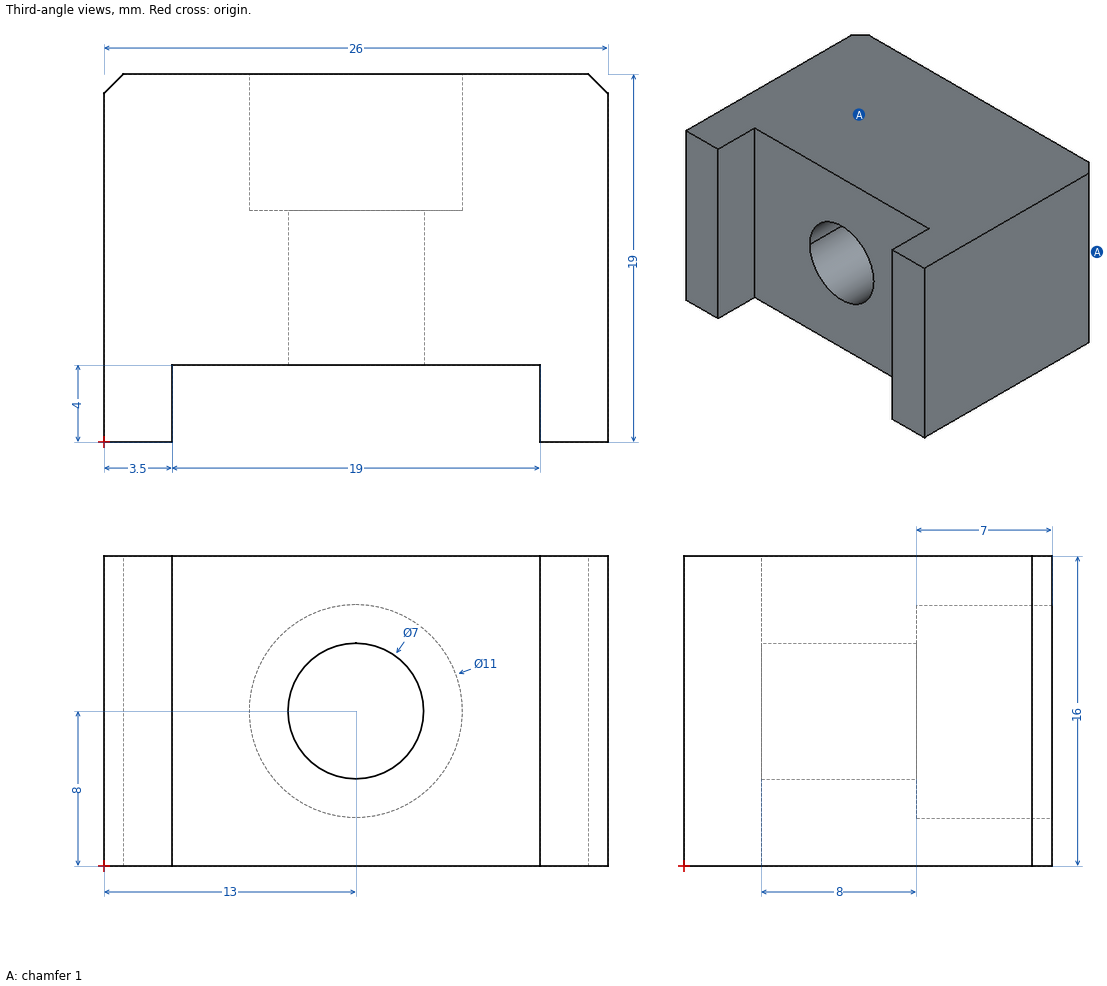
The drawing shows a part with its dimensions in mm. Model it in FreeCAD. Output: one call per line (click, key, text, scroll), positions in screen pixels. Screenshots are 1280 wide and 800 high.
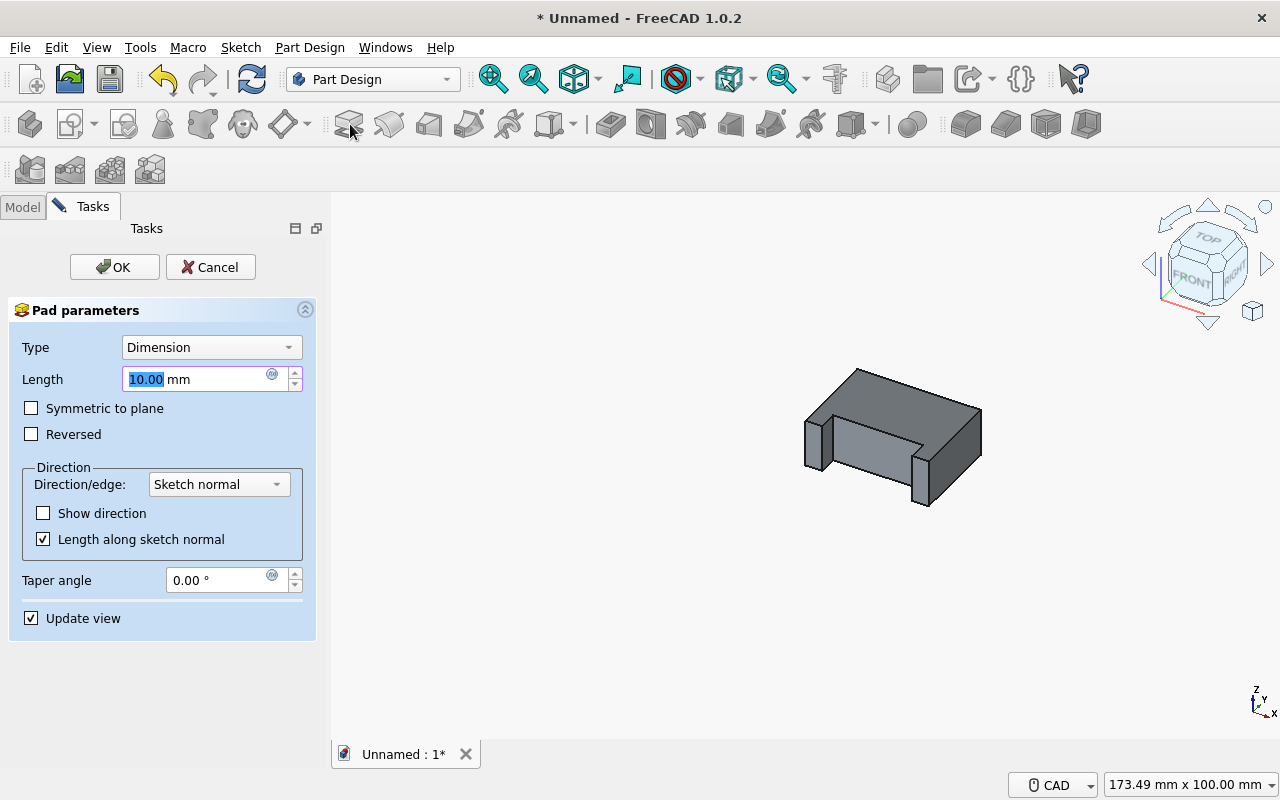
text(16)
key(Tab)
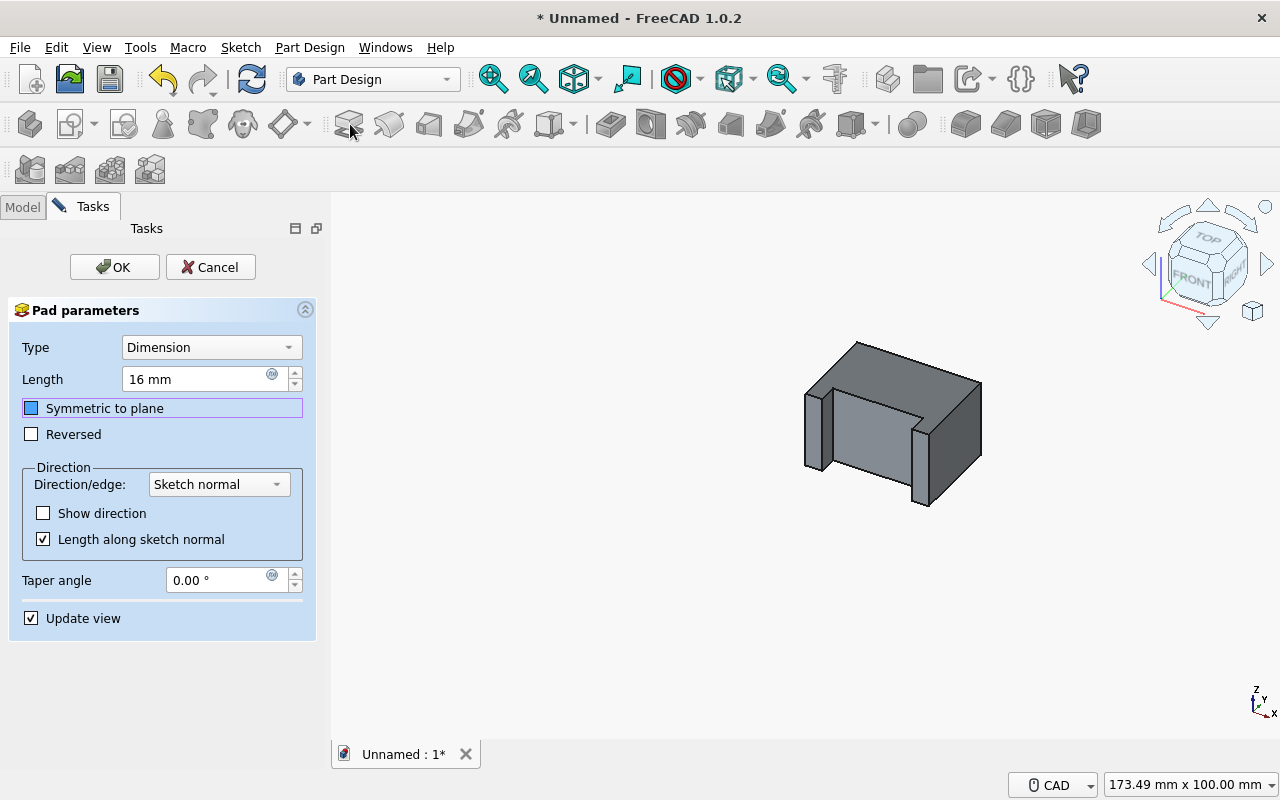
click(115, 267)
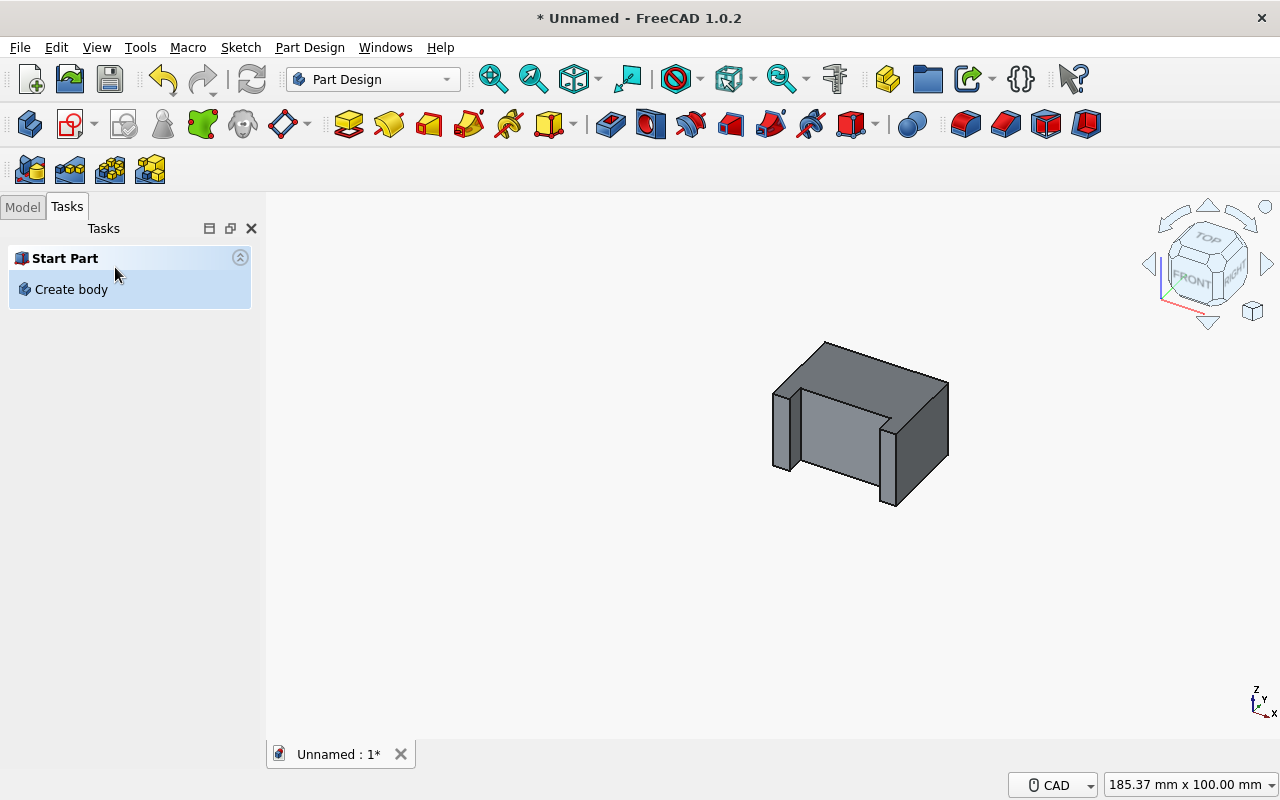
click(494, 80)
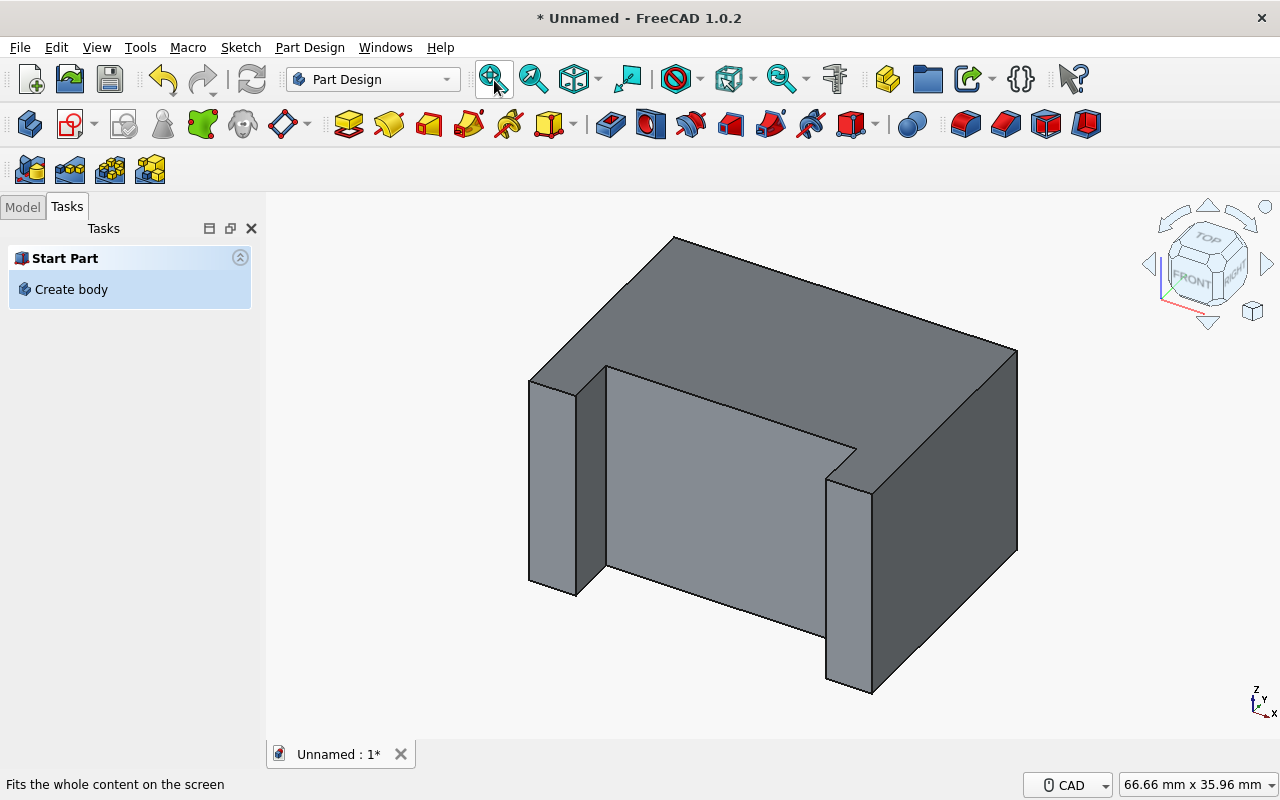
key(4)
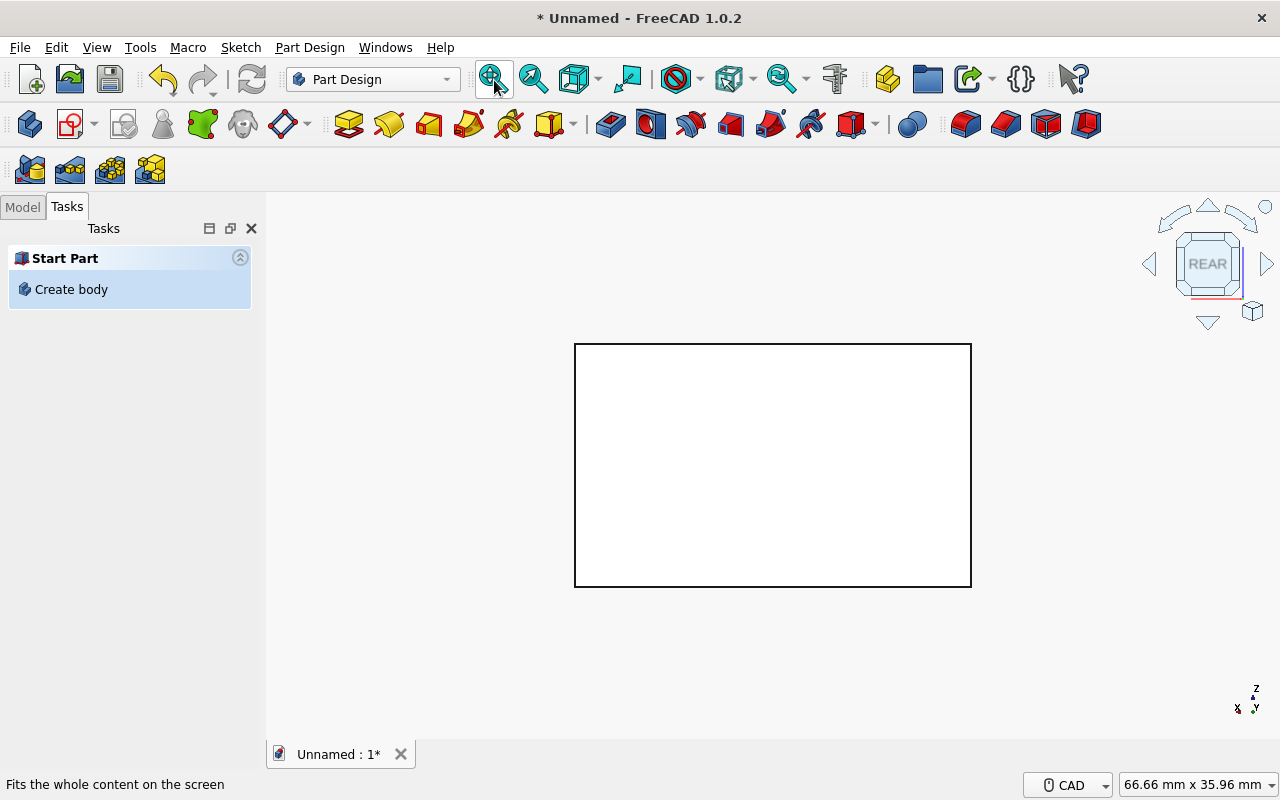
key(v)
key(f)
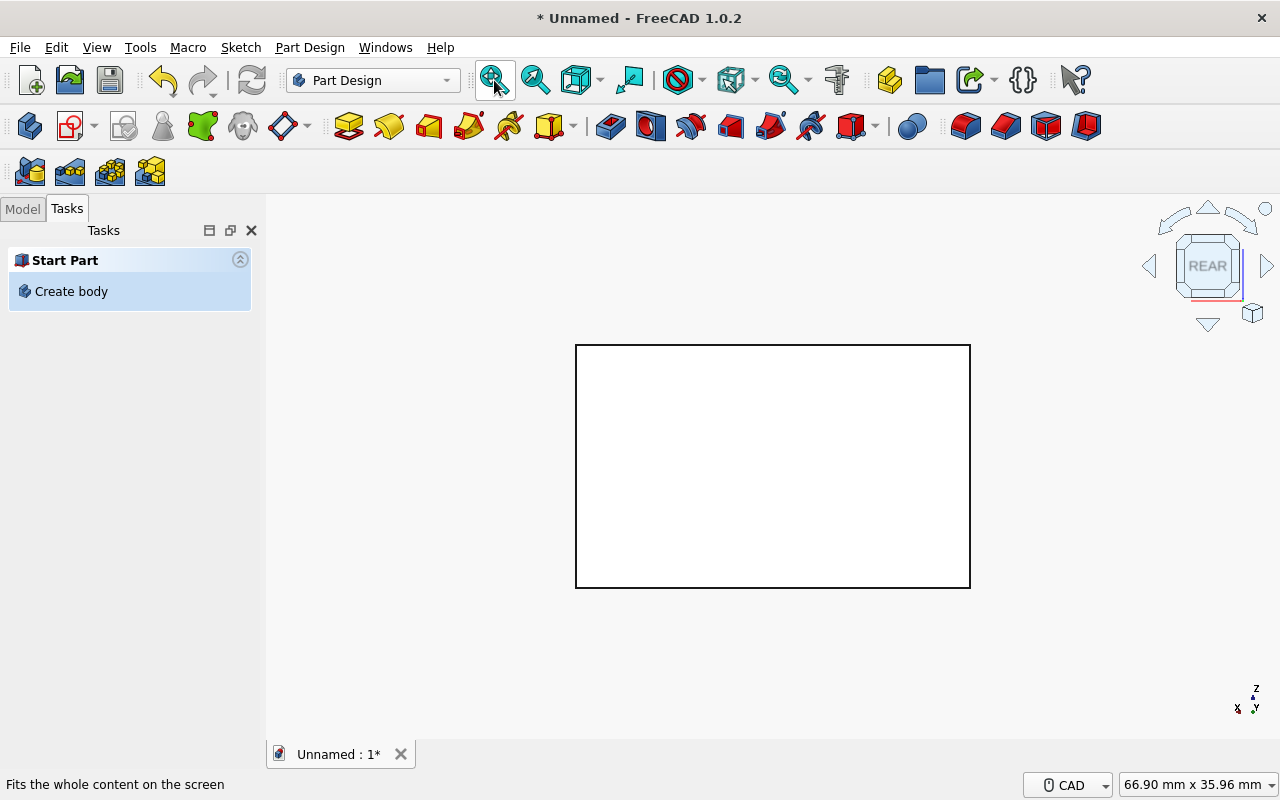
click(717, 466)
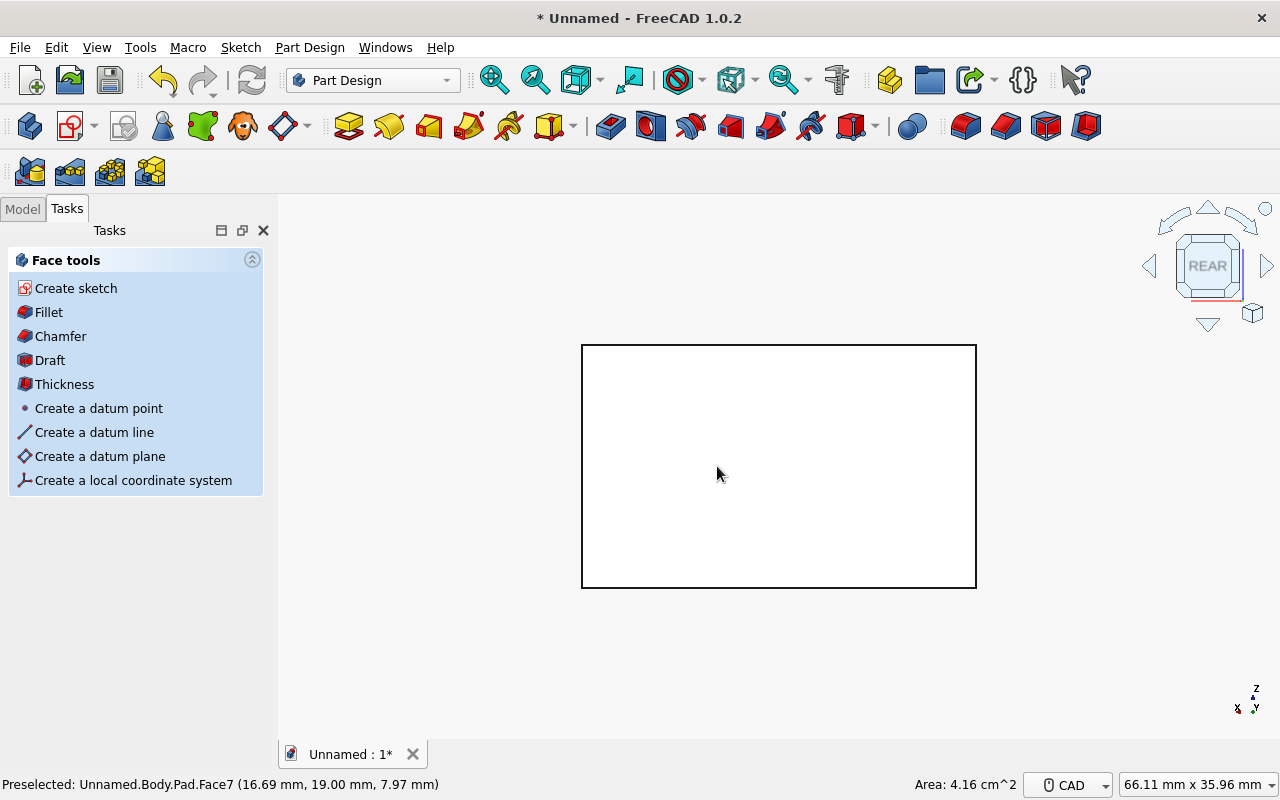
click(70, 126)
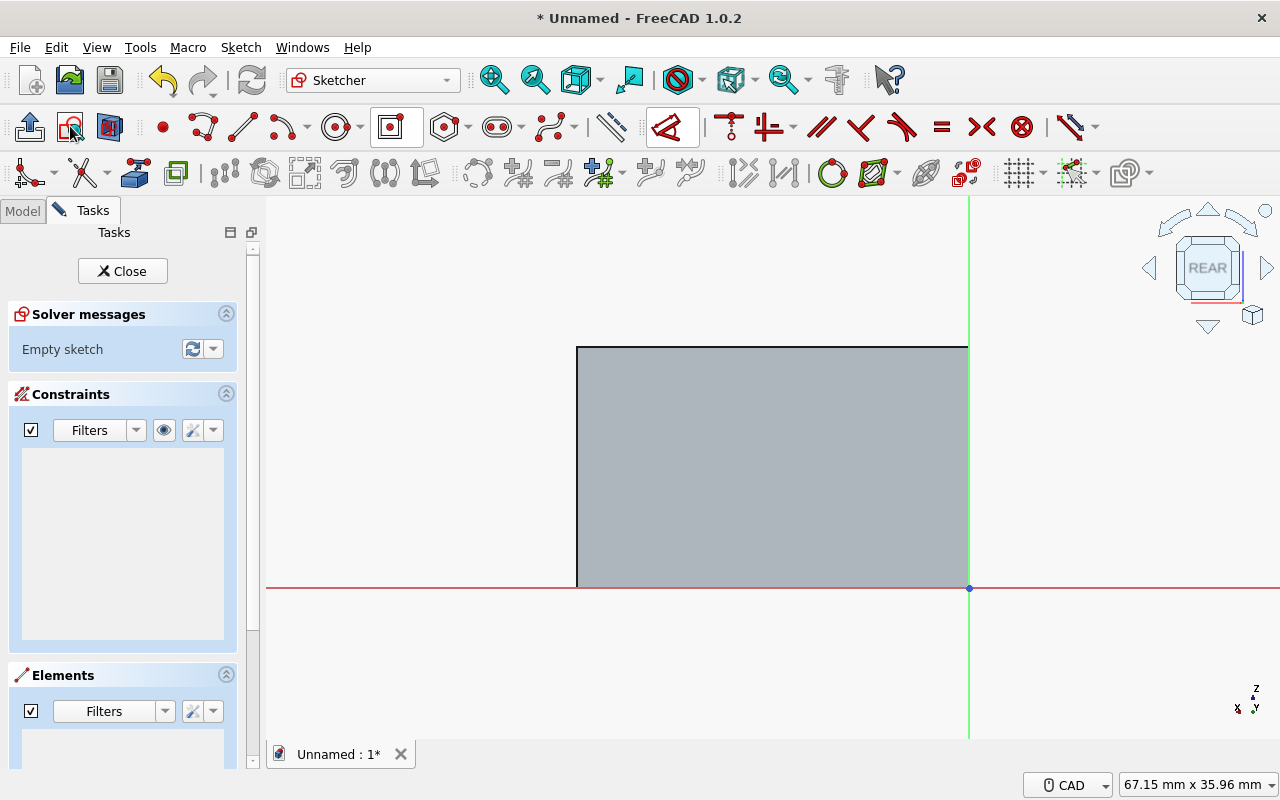
scroll(982, 509, up, 3)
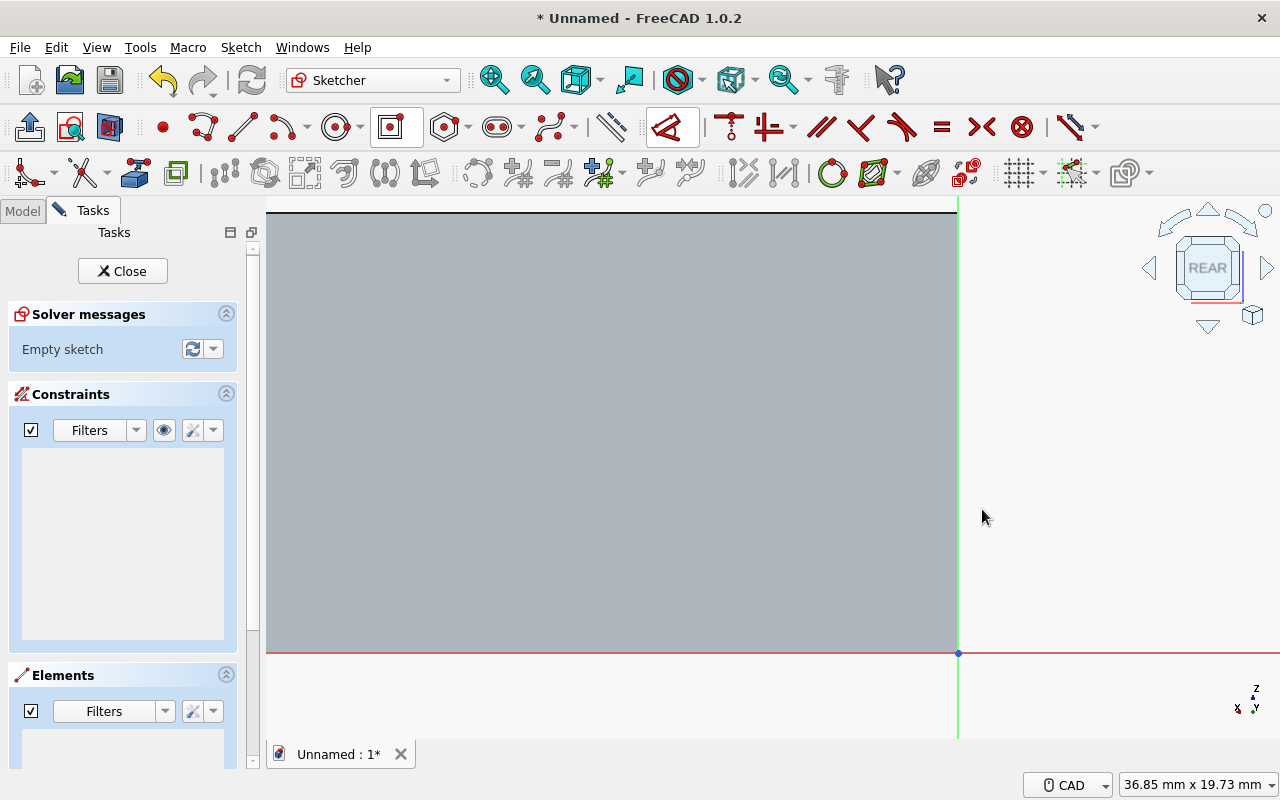
key(g)
key(c)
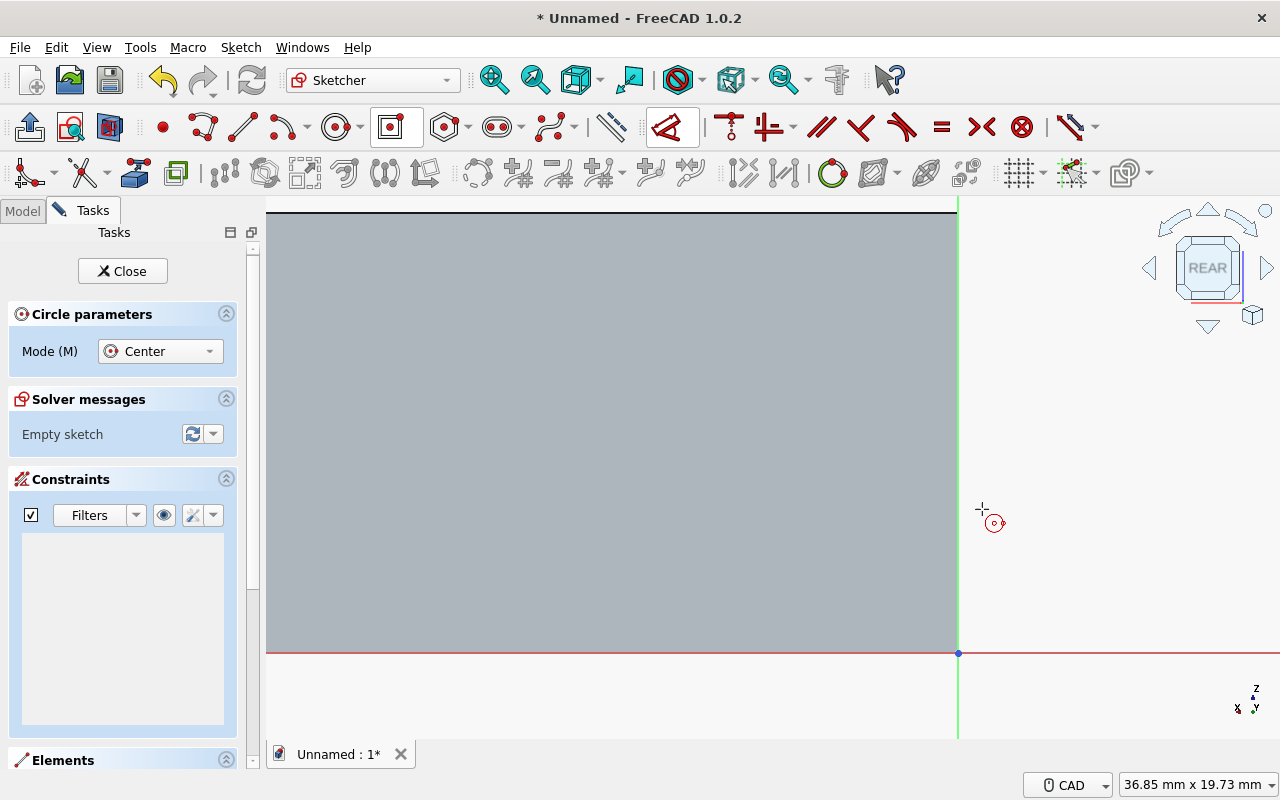
click(601, 433)
move(708, 326)